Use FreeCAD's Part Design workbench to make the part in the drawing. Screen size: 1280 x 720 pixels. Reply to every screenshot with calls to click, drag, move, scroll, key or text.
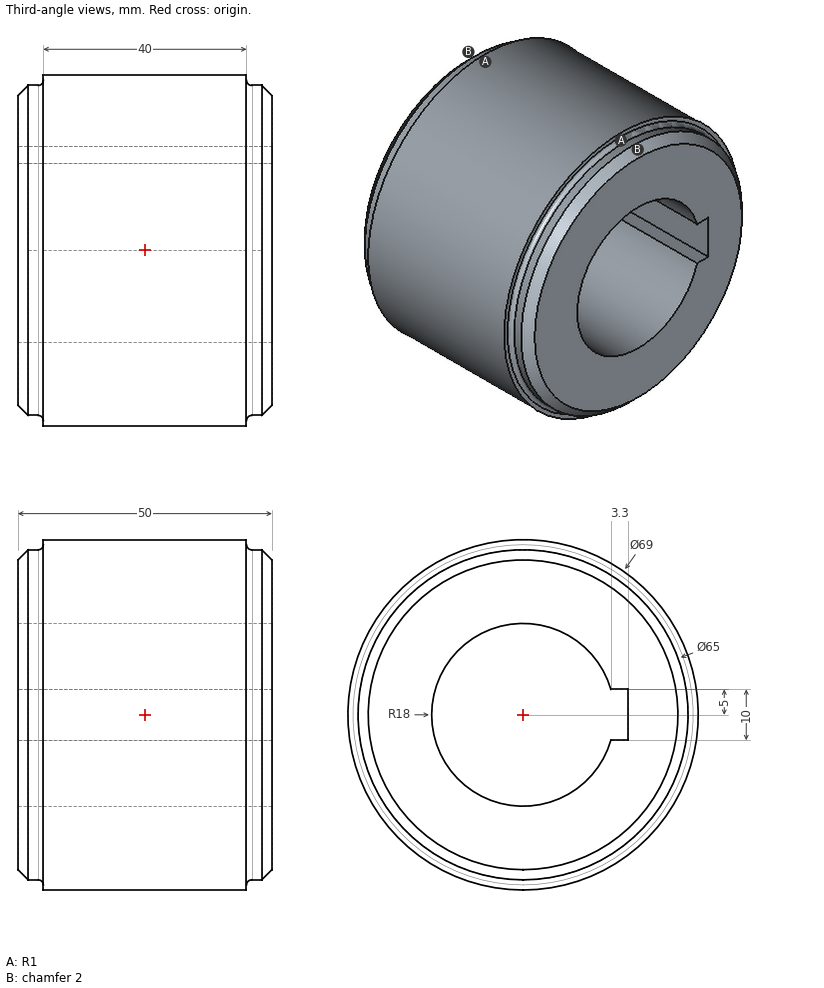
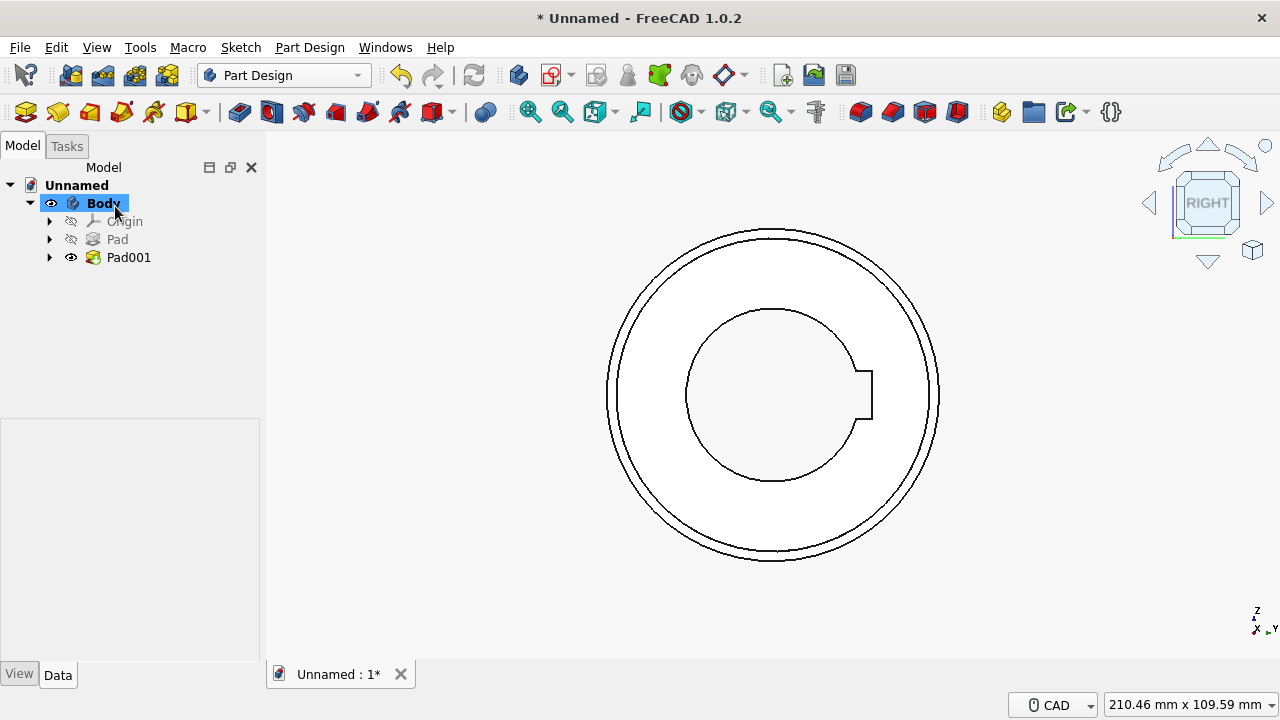
key(5)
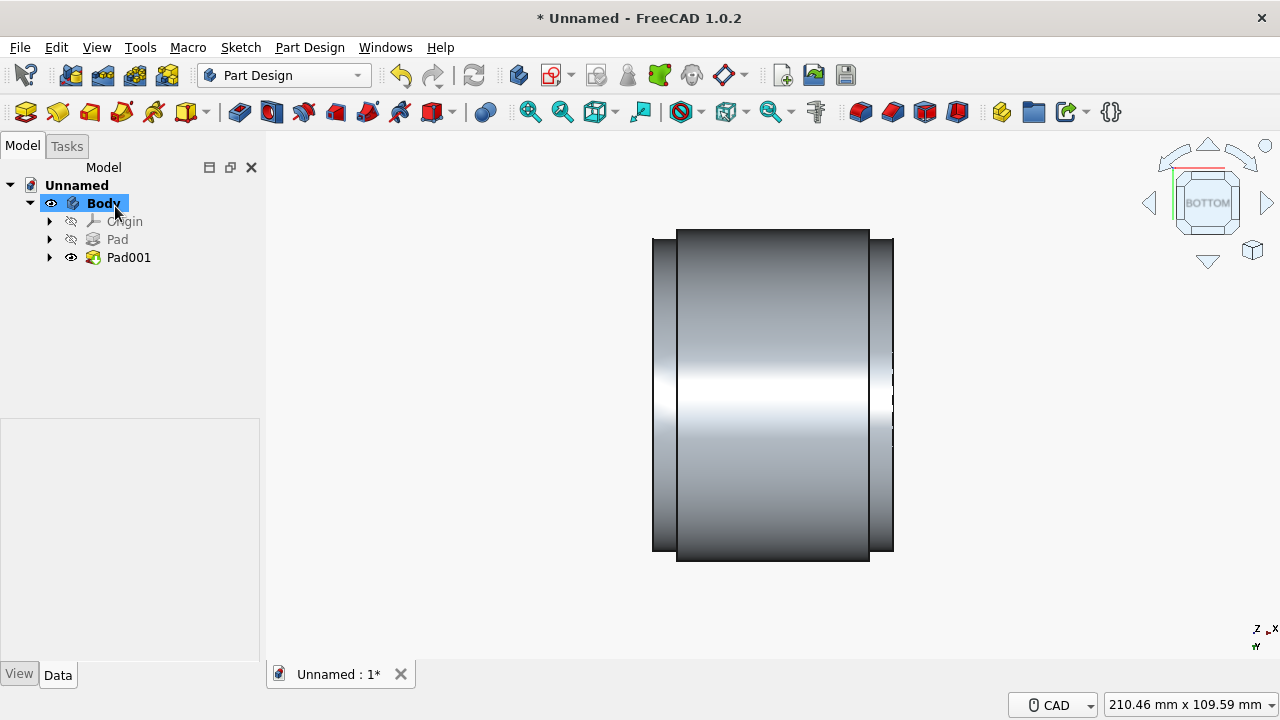
key(4)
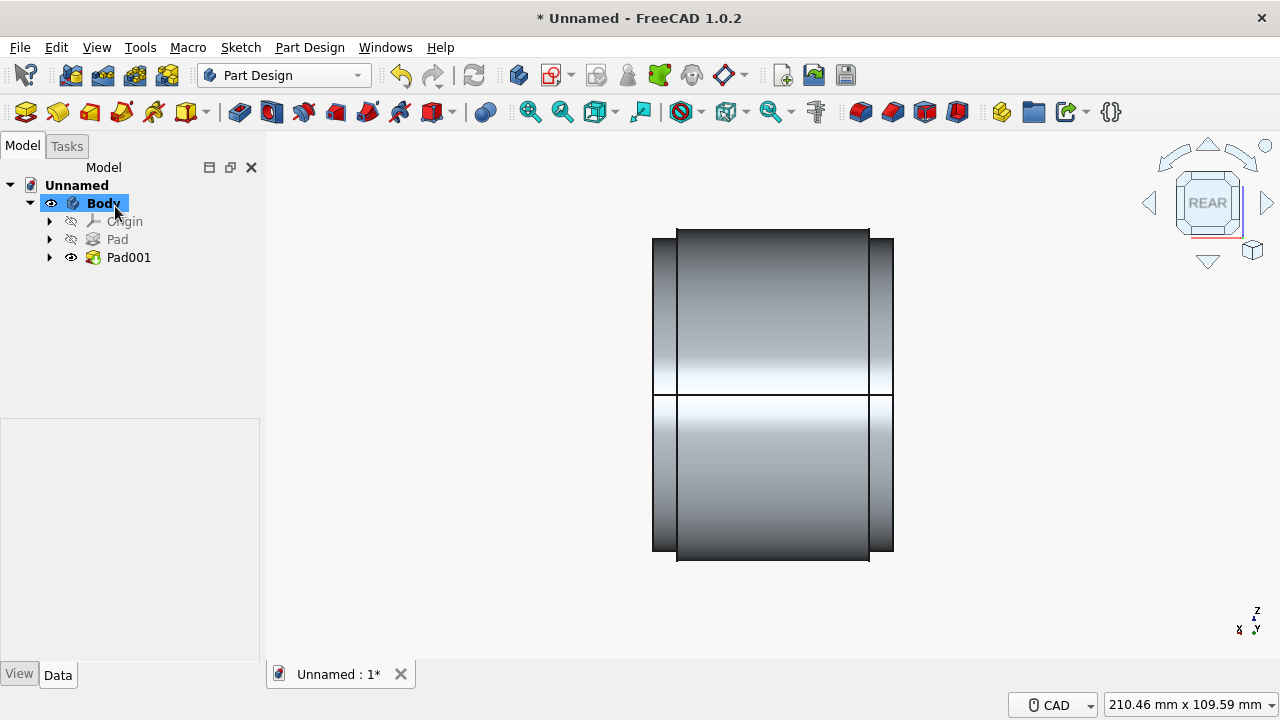
key(6)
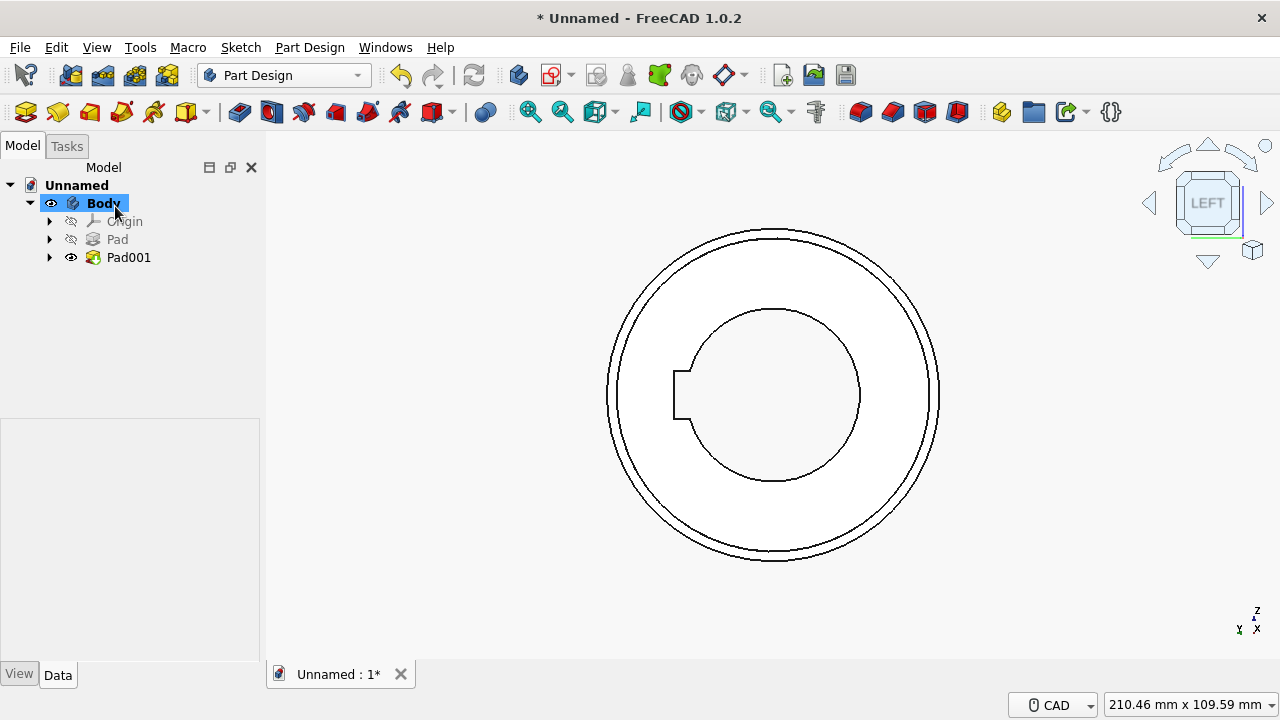
key(v)
key(3)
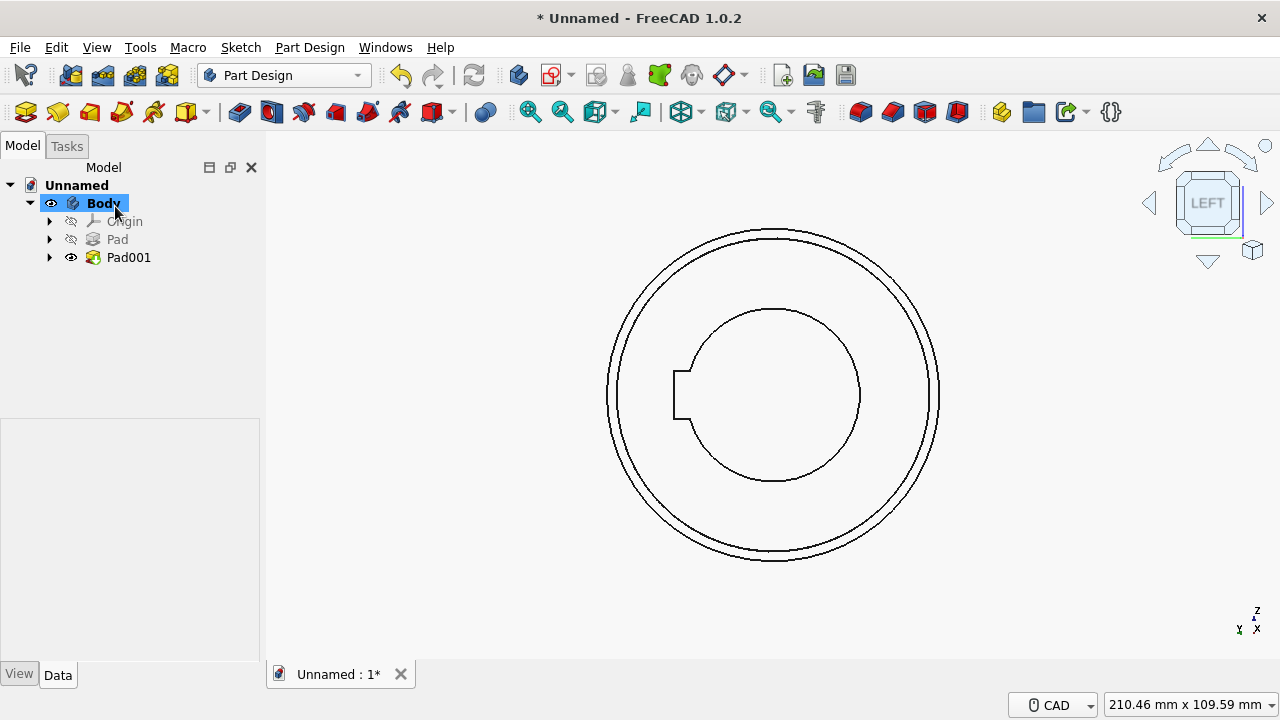
key(0)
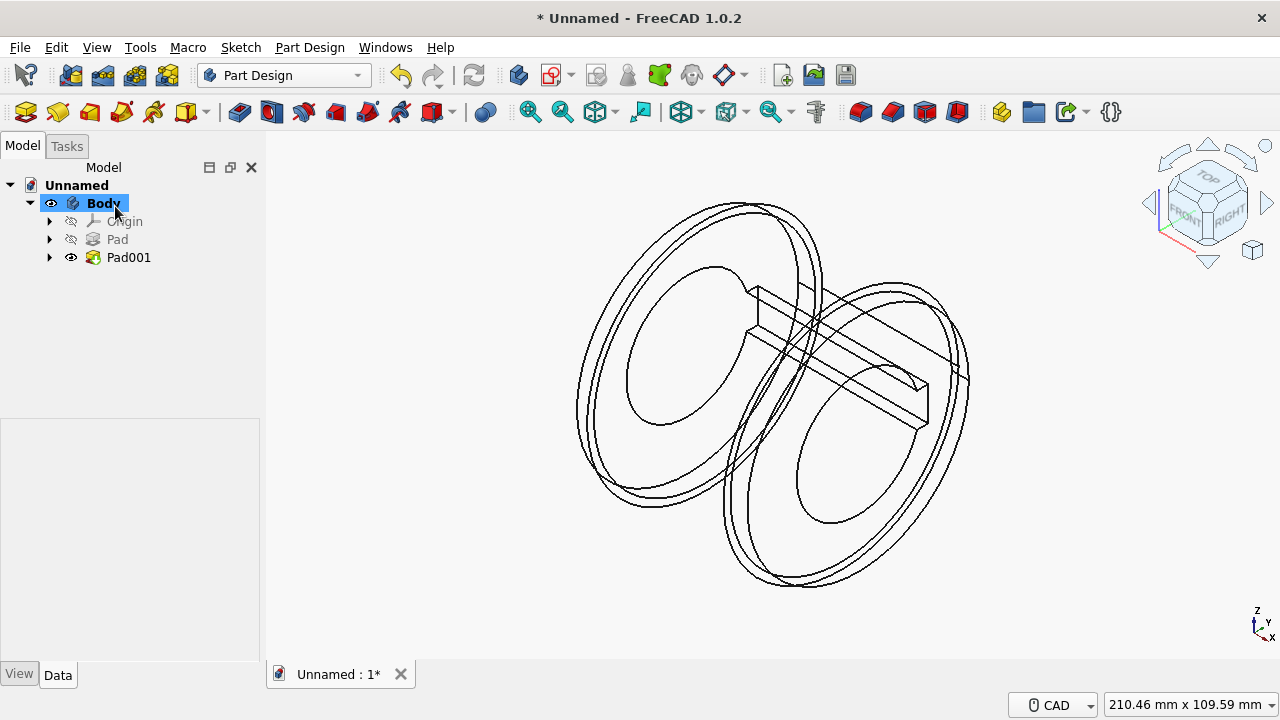
click(594, 419)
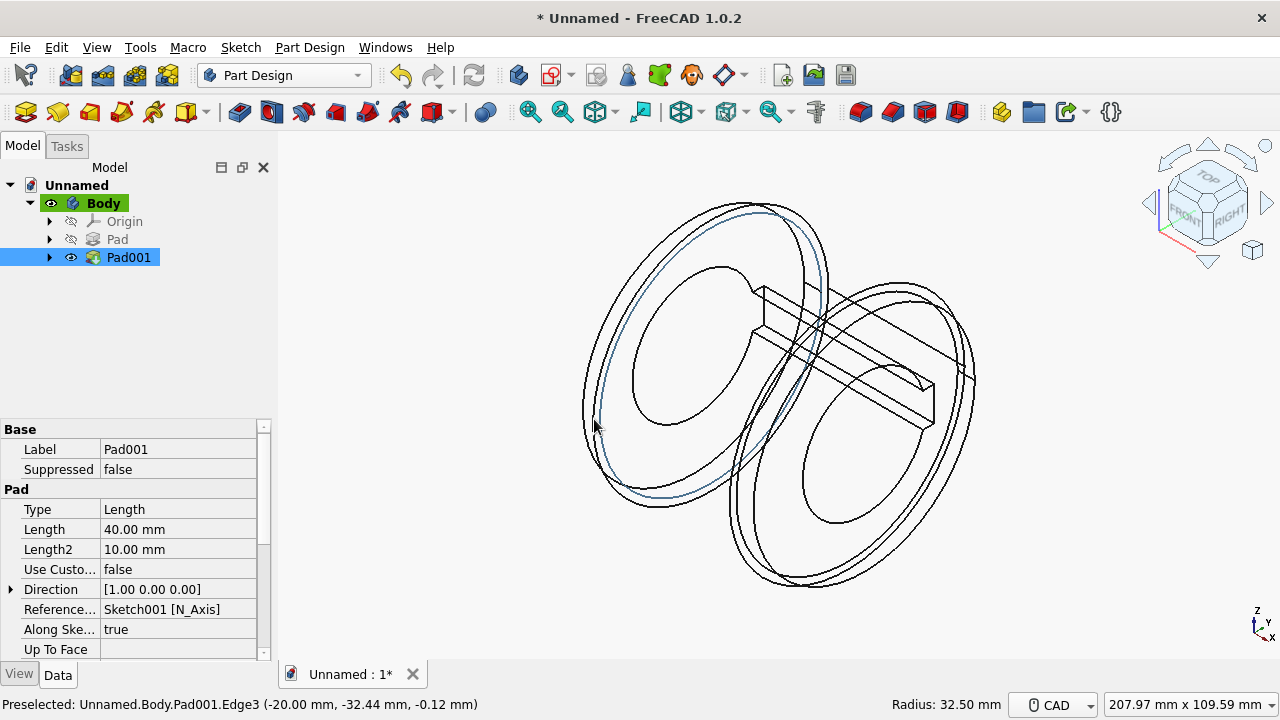
click(736, 497, ctrl)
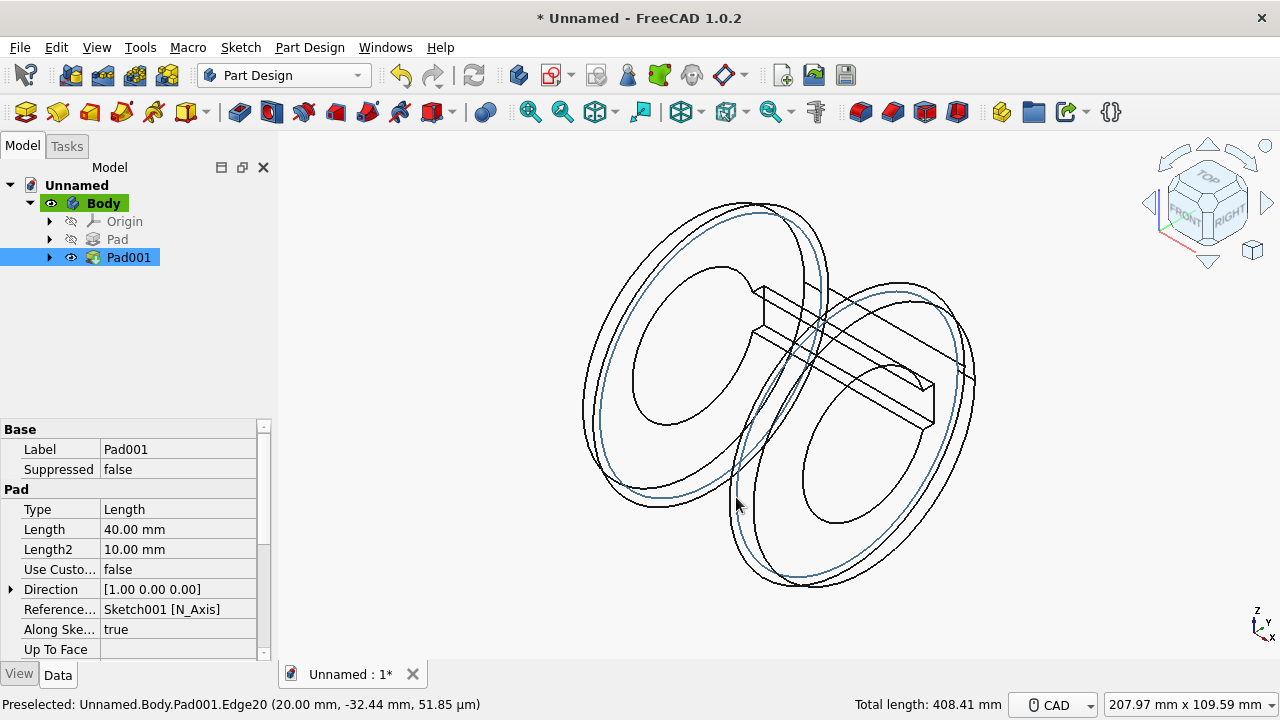
key(v)
key(1)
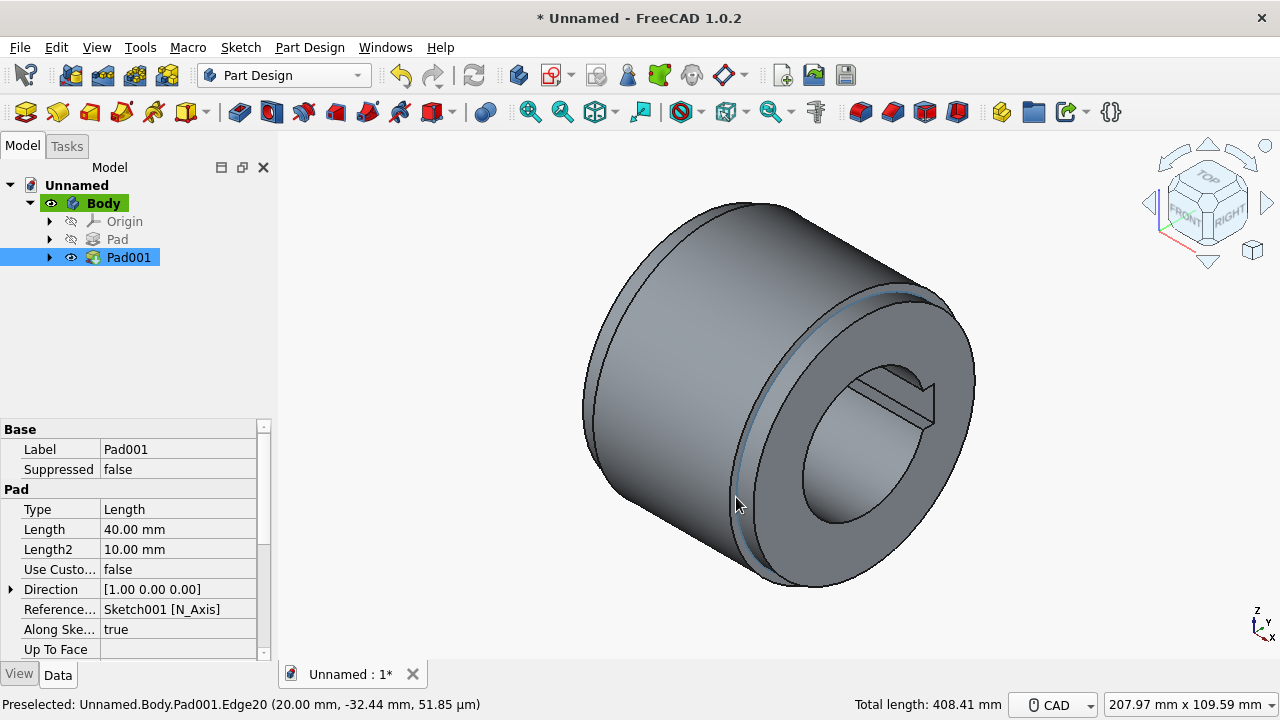
click(862, 112)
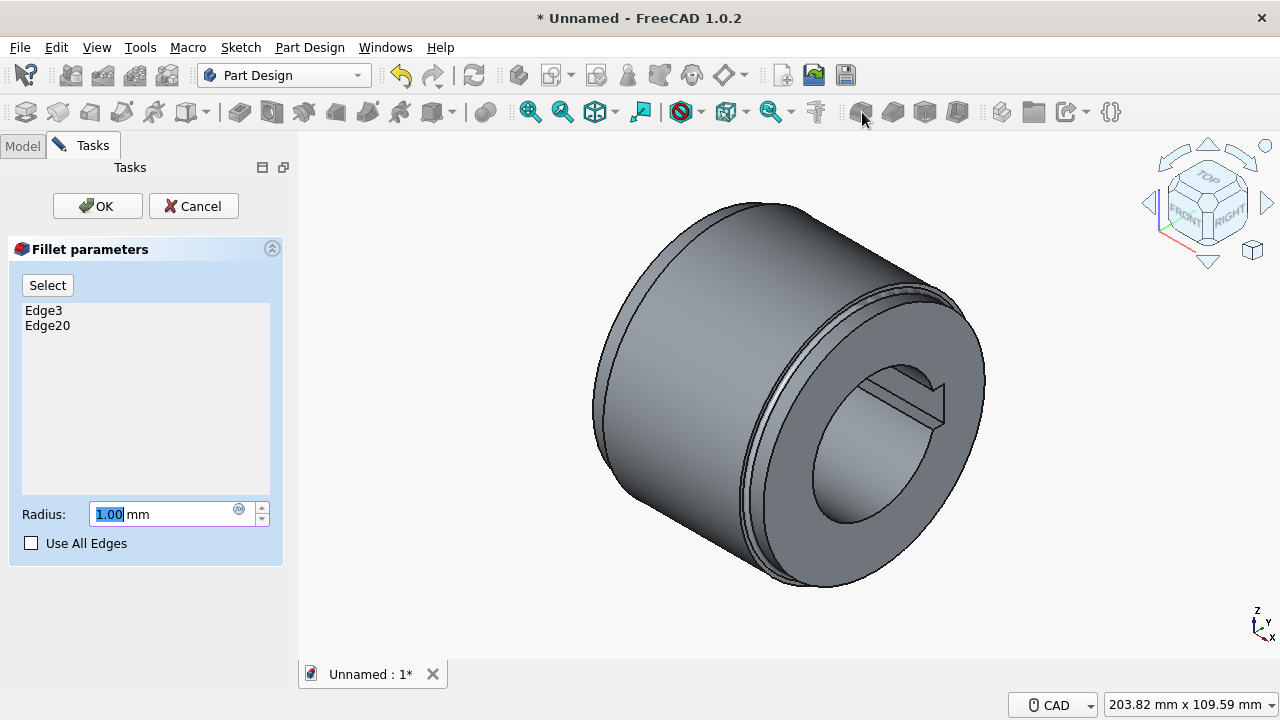
text(1)
key(Tab)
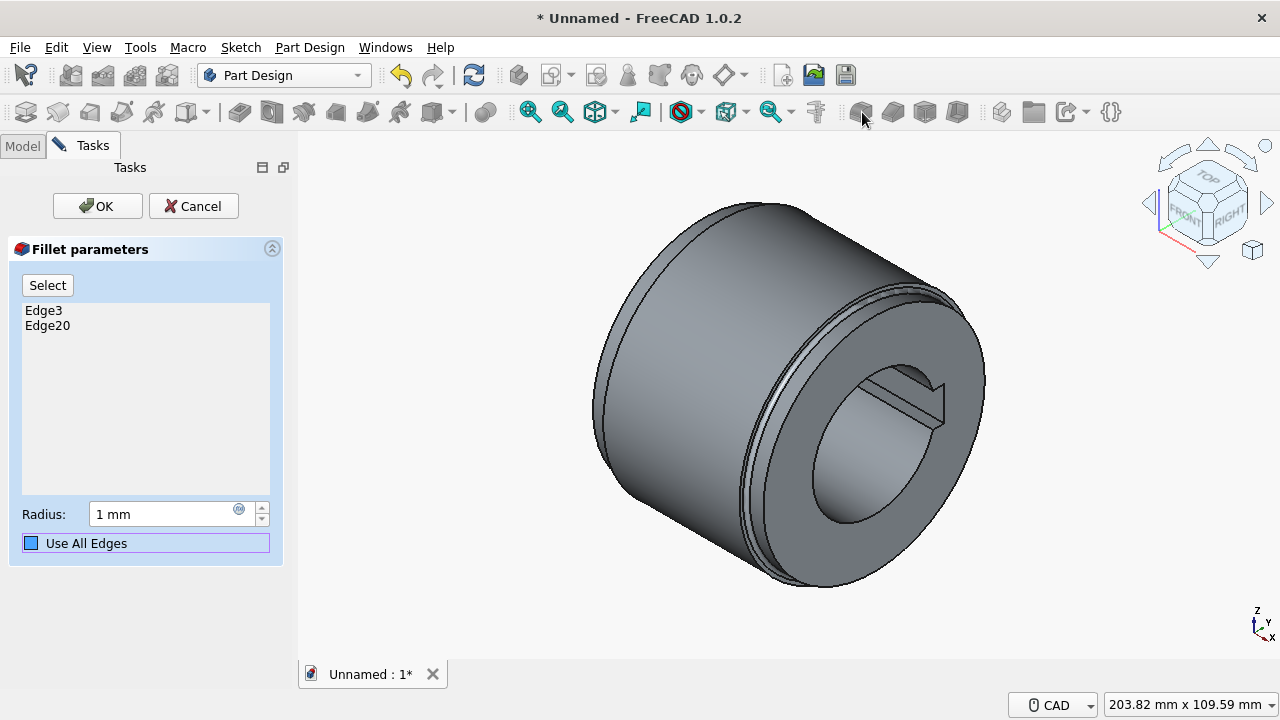
click(98, 206)